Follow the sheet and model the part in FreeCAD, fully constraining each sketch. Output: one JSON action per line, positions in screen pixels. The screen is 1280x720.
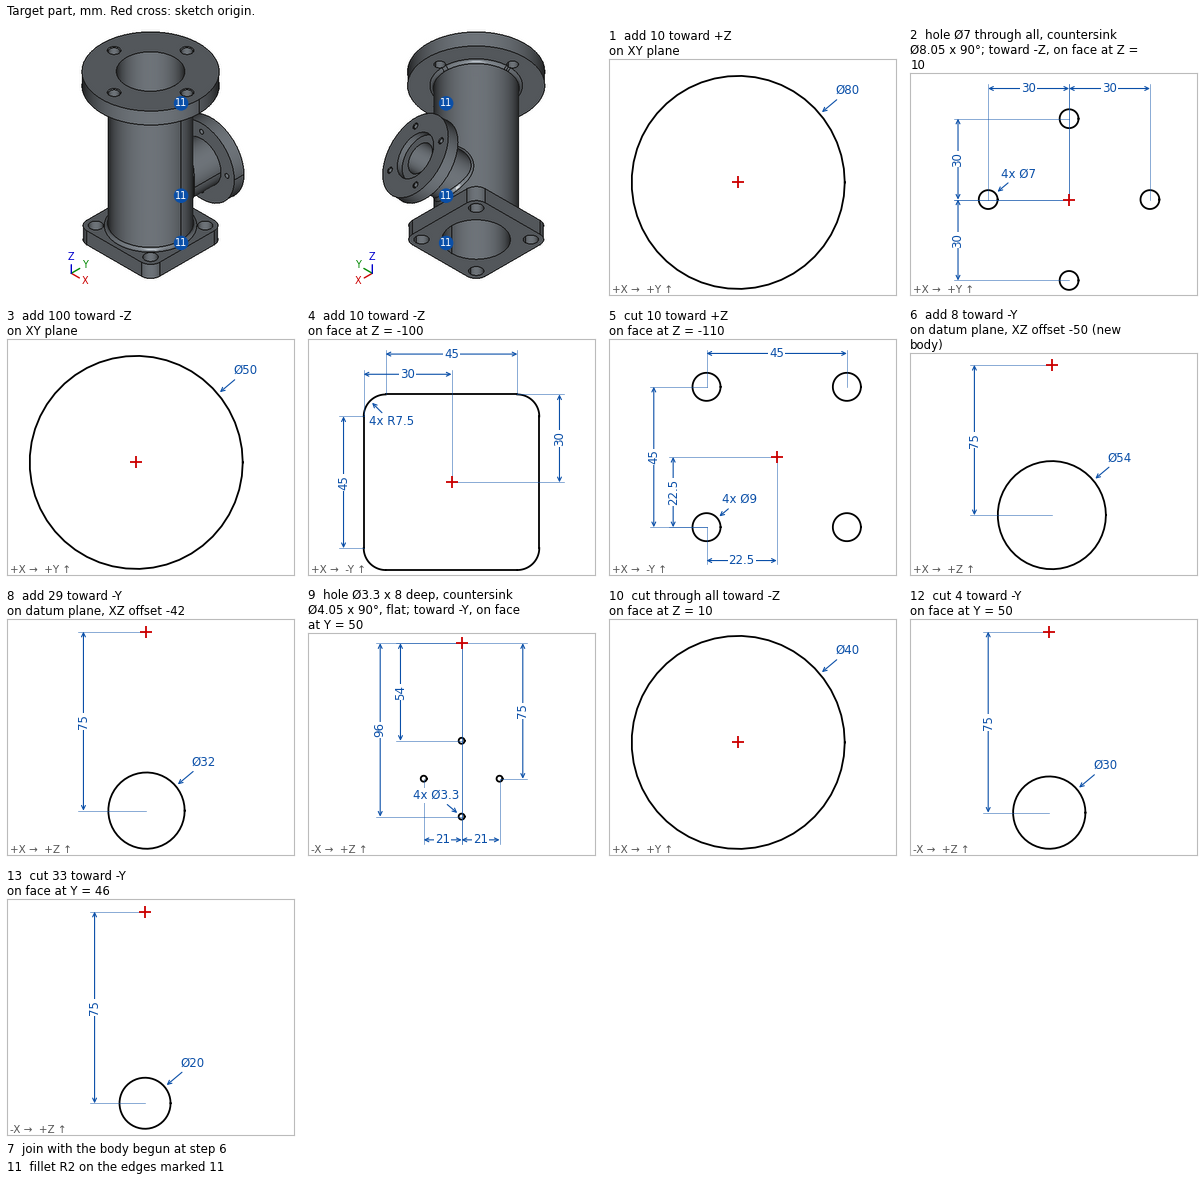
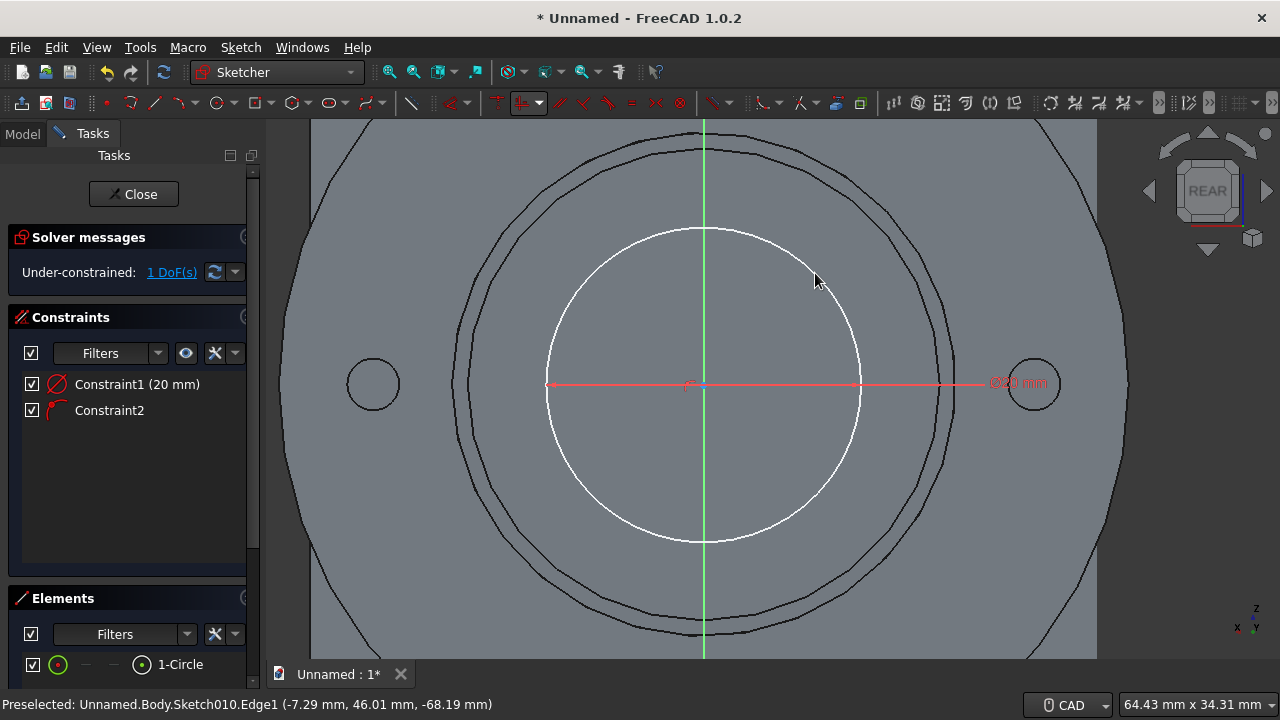
{"action": "left_click", "coordinate": [450, 104]}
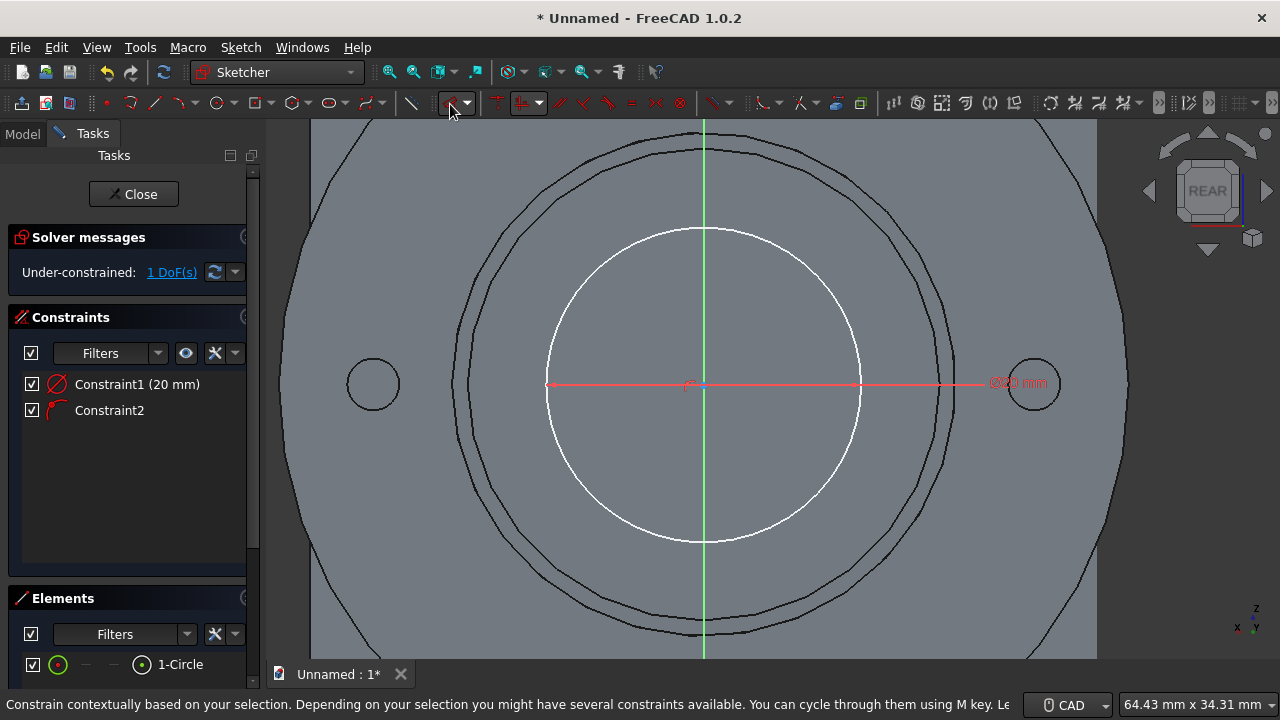
{"action": "left_click", "coordinate": [704, 385]}
{"action": "left_click", "coordinate": [738, 266]}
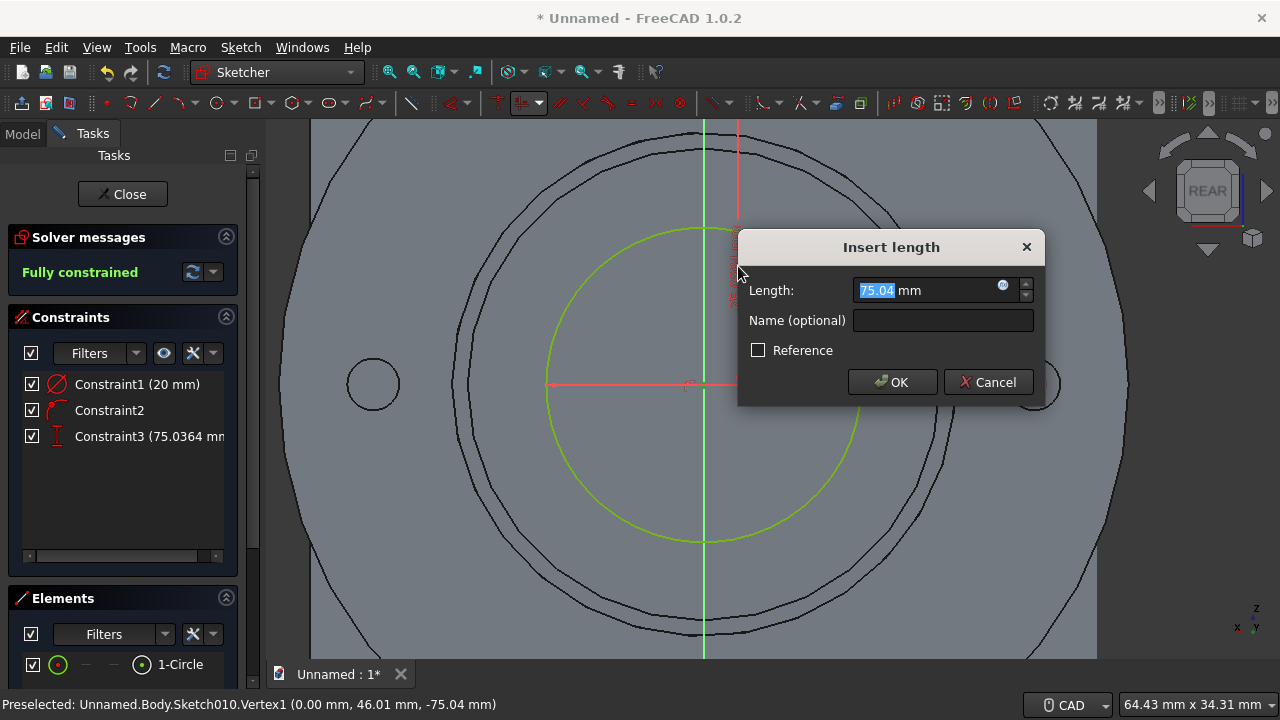
{"action": "type", "text": "75"}
{"action": "key", "text": "Return"}
{"action": "key", "text": "Escape"}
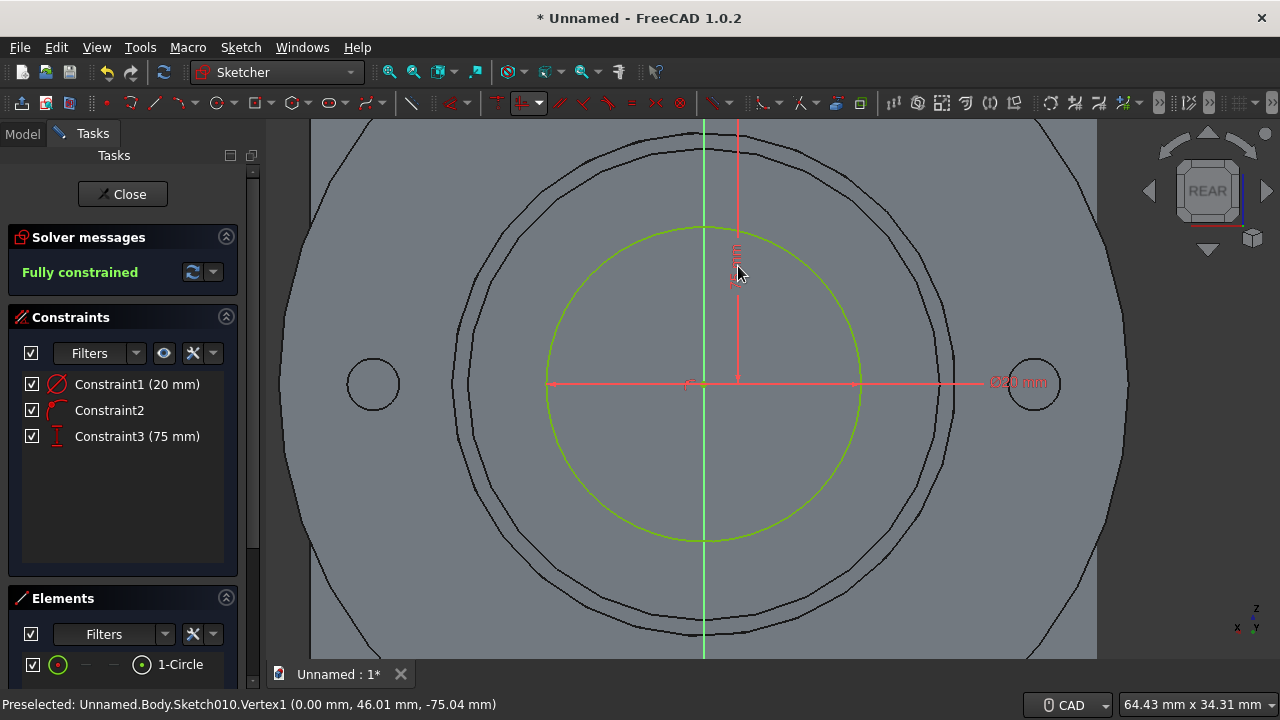
{"action": "left_click", "coordinate": [123, 194]}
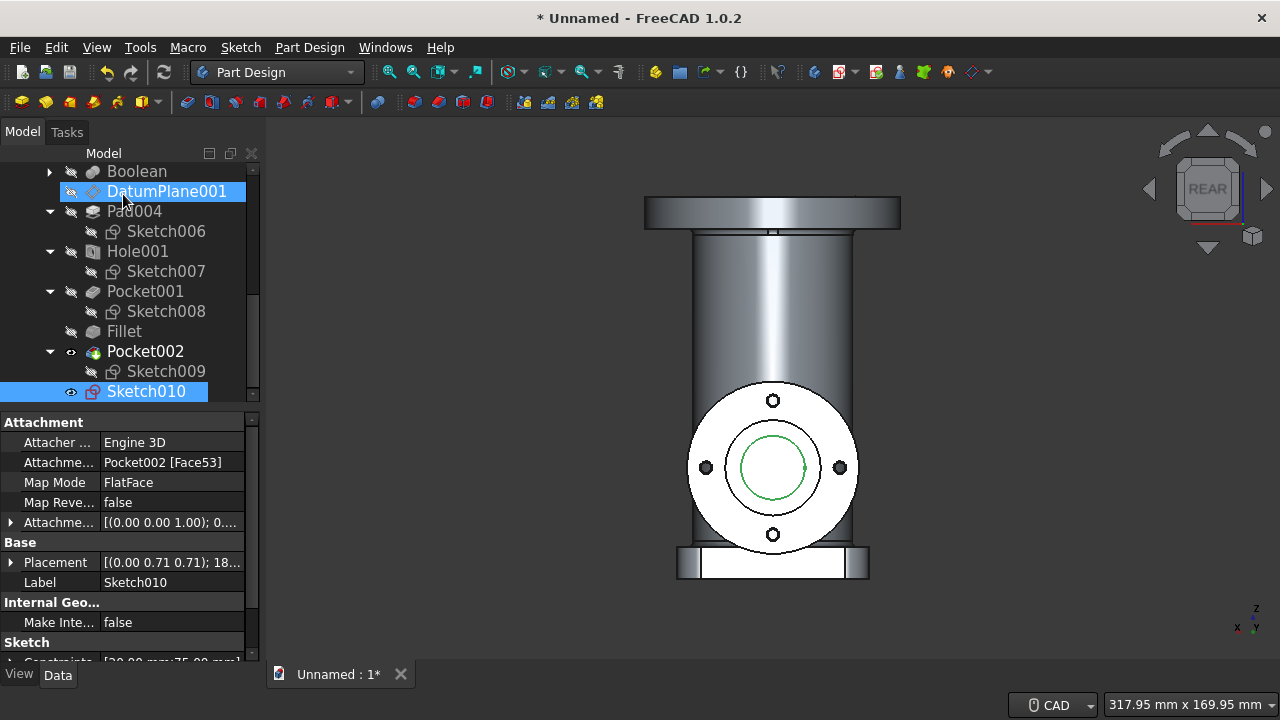
{"action": "left_click", "coordinate": [188, 102]}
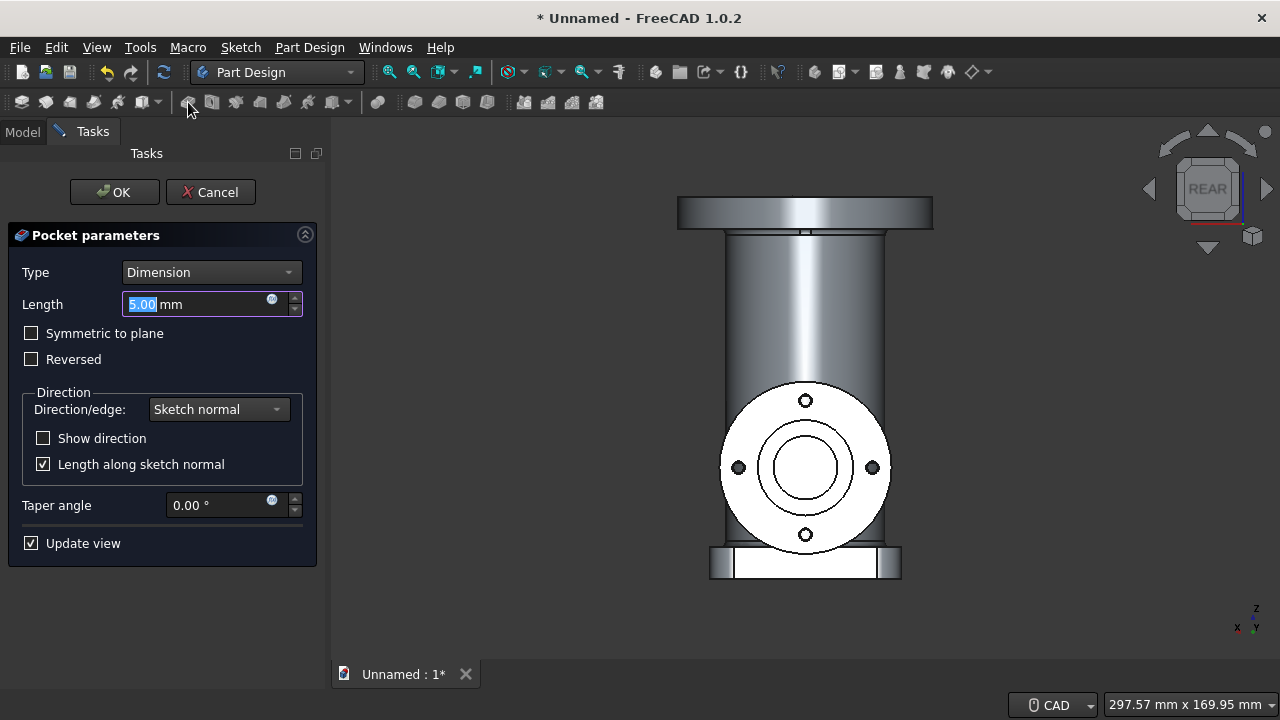
{"action": "type", "text": "33"}
{"action": "key", "text": "Tab"}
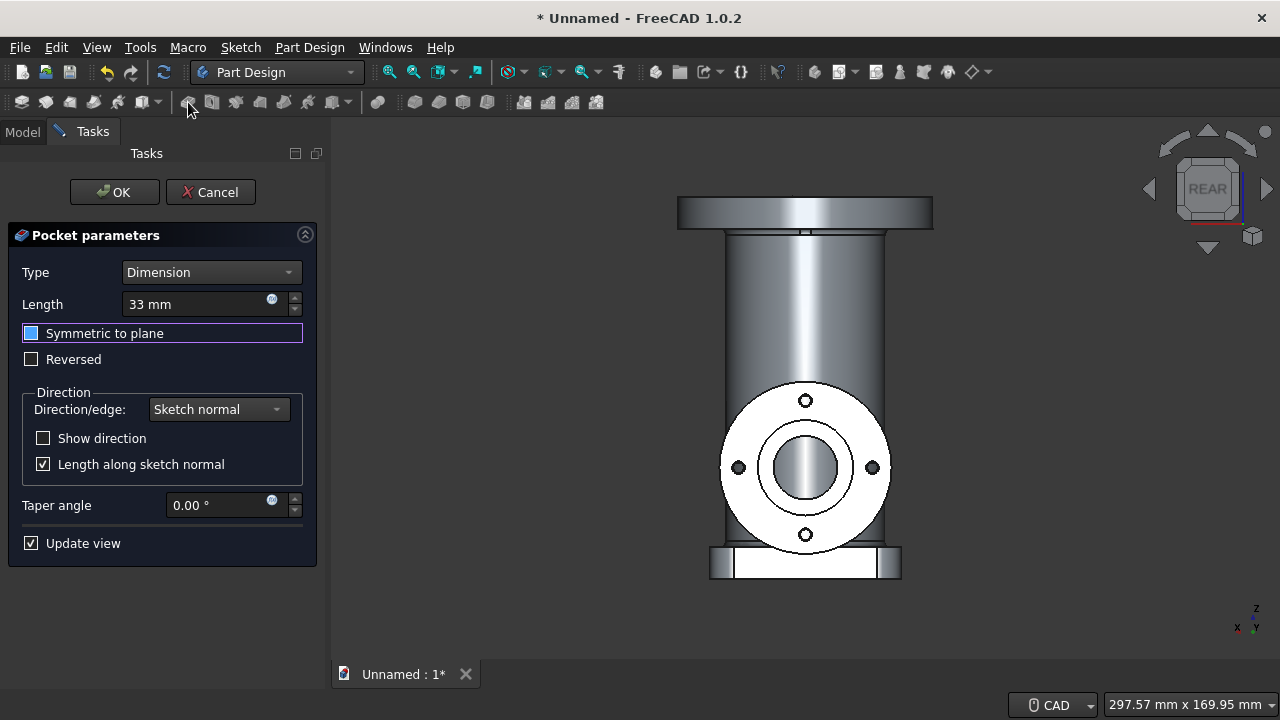
{"action": "left_click", "coordinate": [115, 192]}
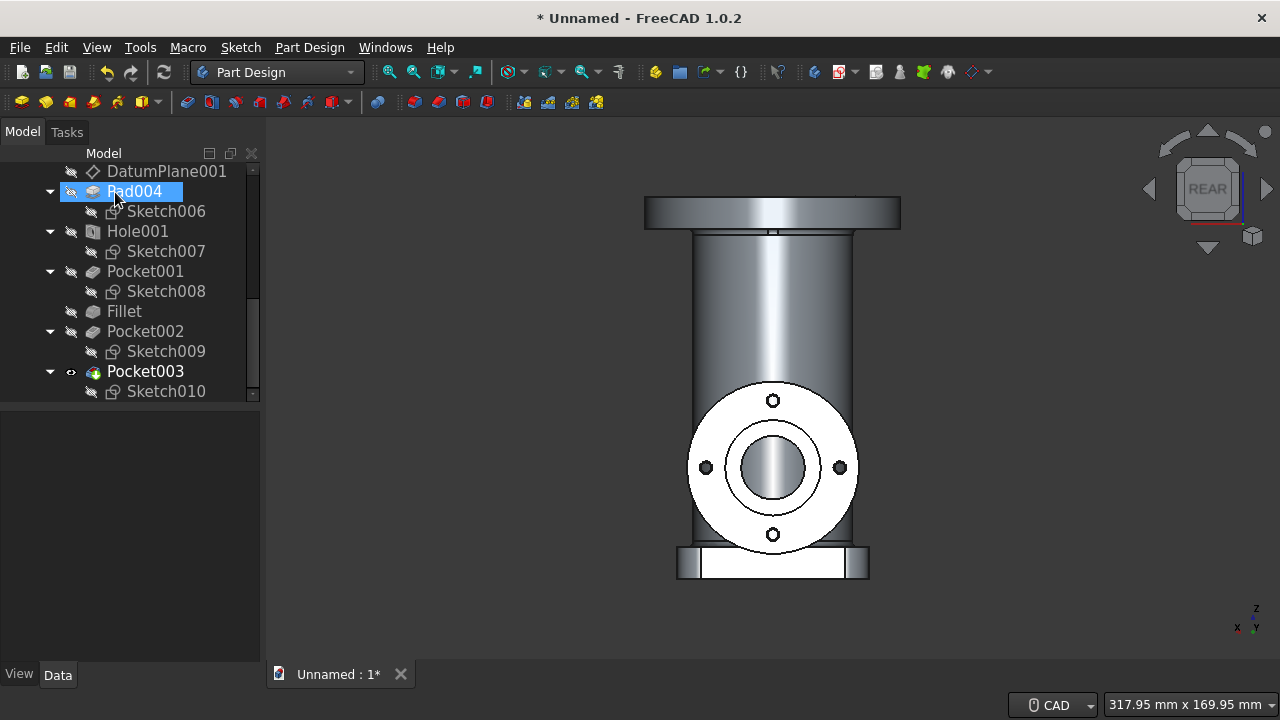
{"action": "key", "text": "0"}